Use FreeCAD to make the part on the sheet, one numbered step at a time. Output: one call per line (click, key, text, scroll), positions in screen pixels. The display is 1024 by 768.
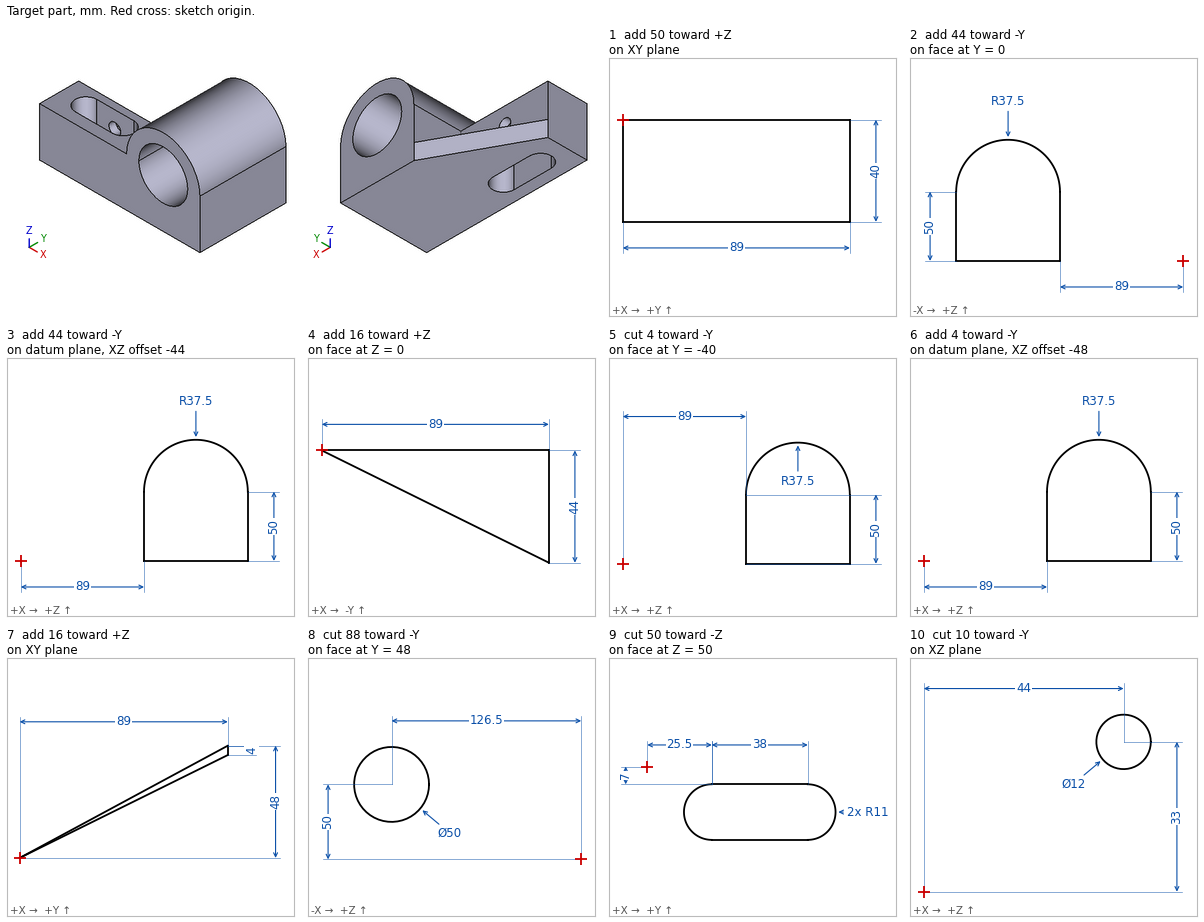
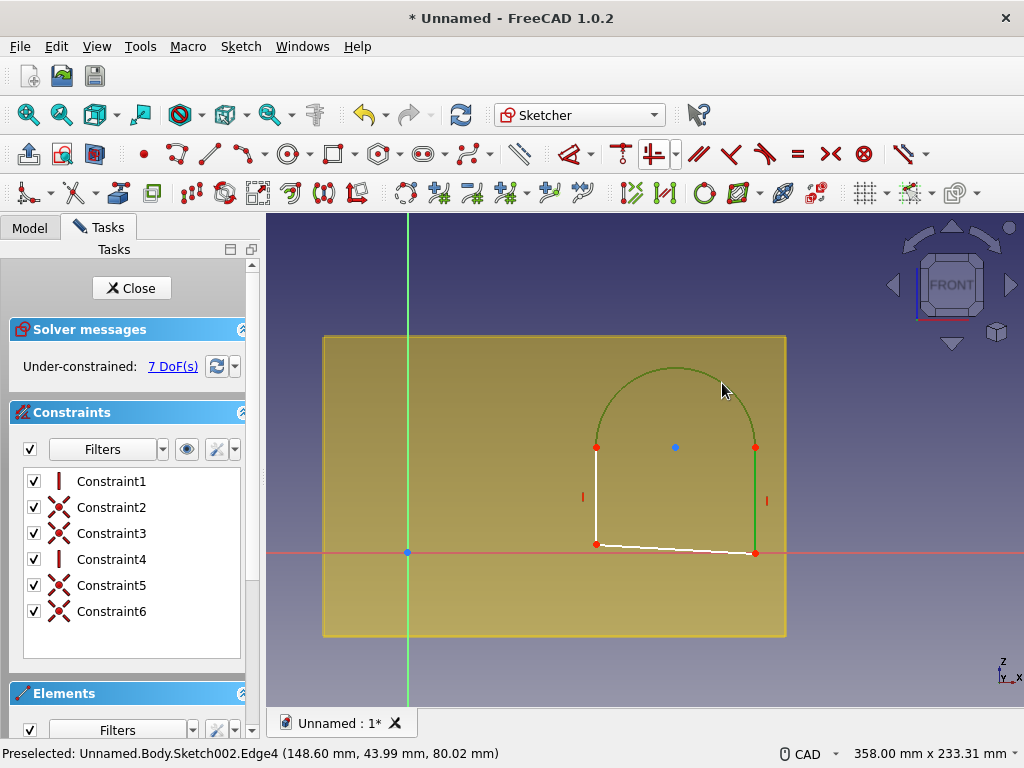
click(765, 154)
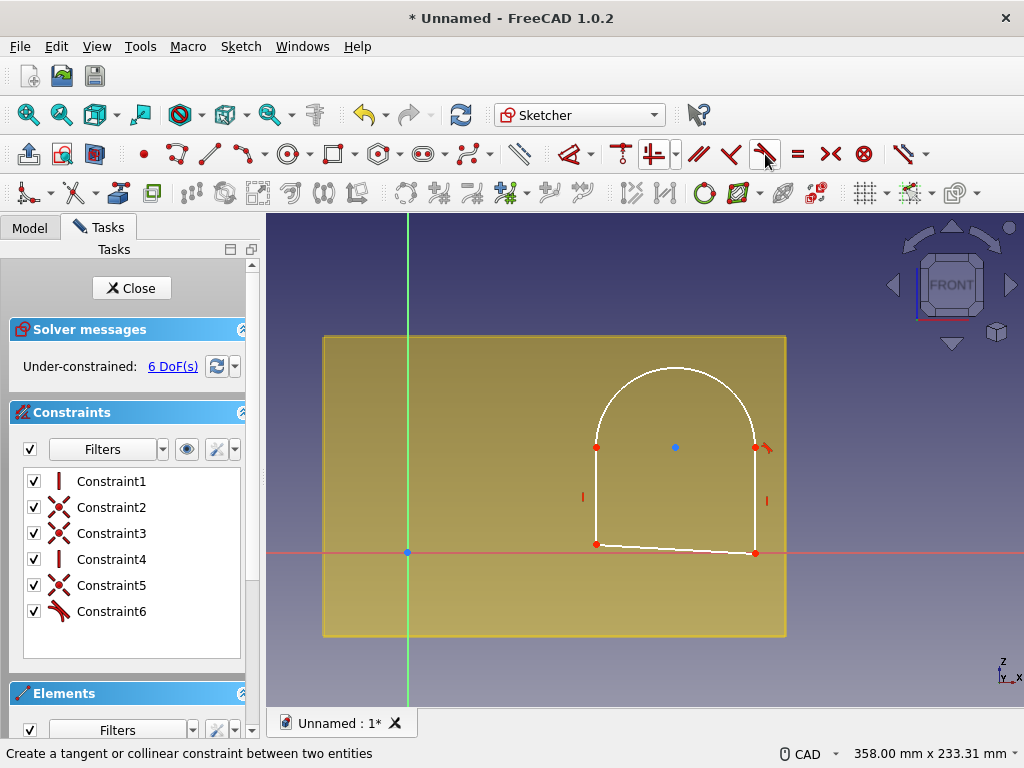
click(596, 516)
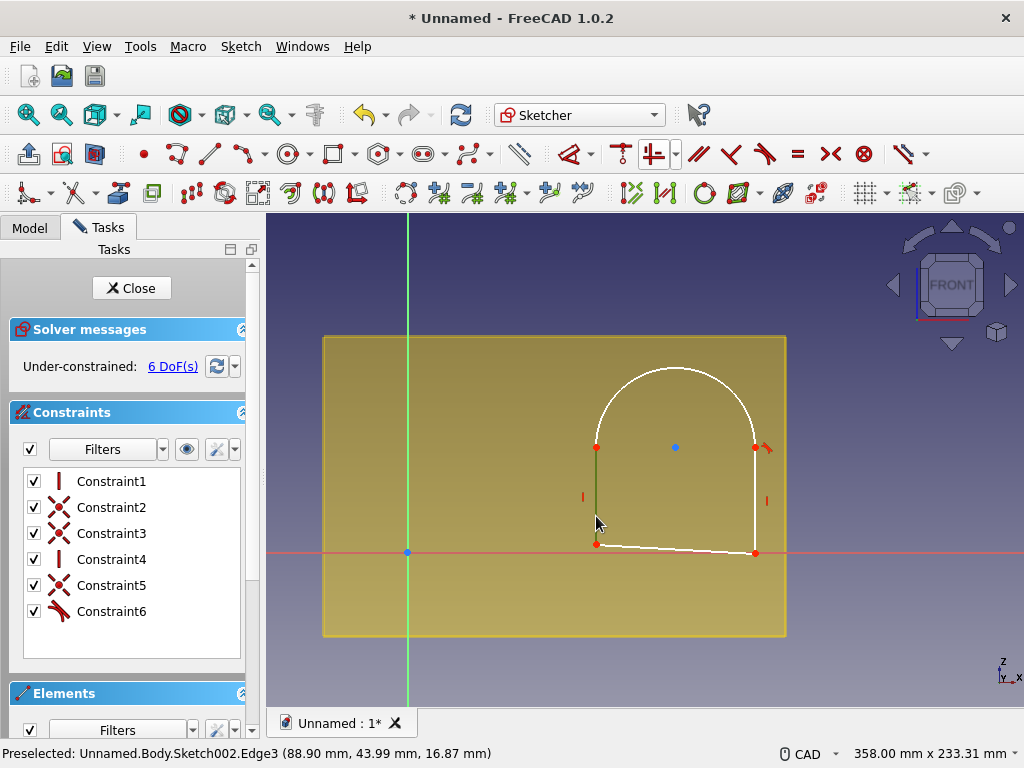
click(722, 383)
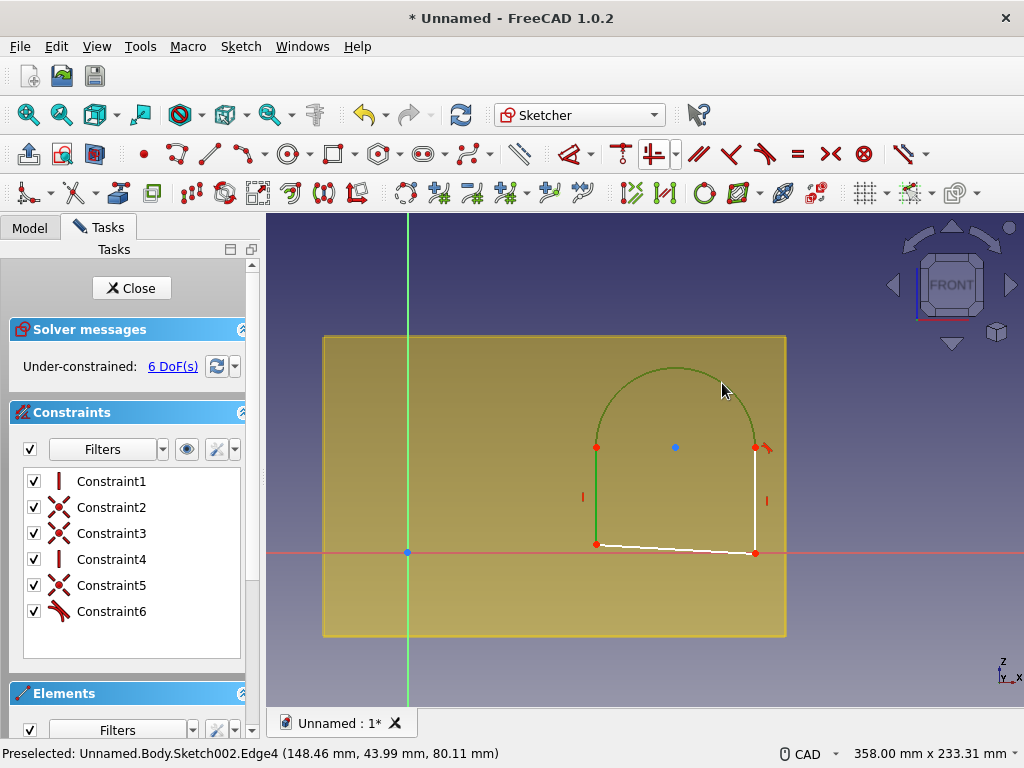
click(765, 154)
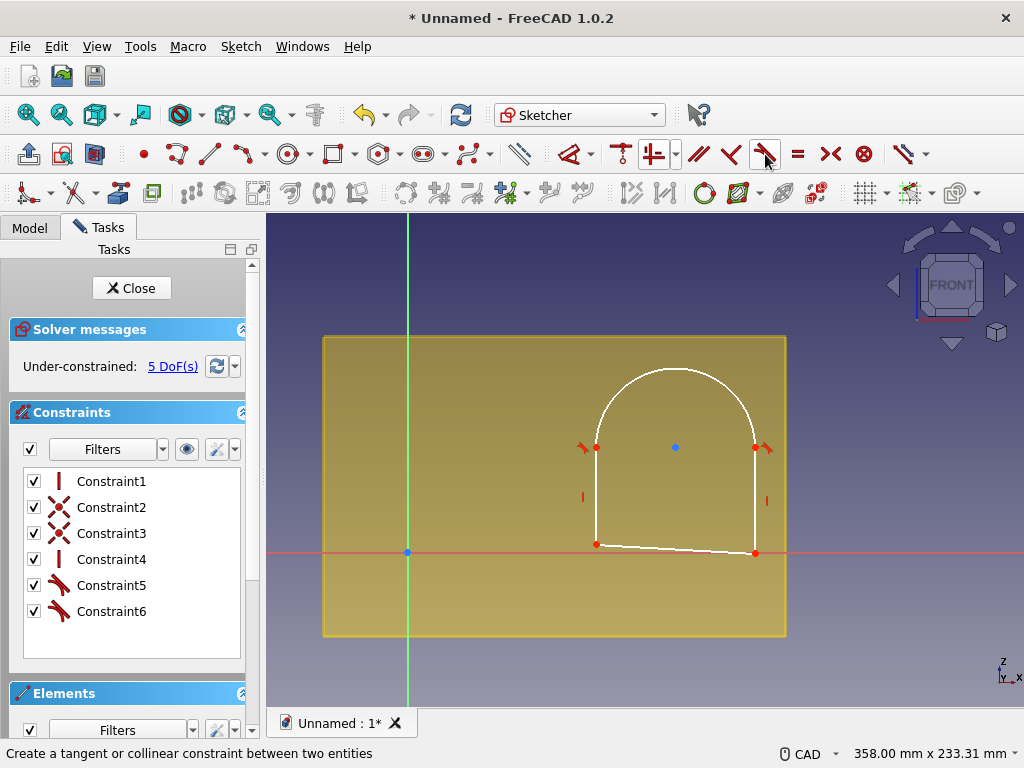
click(707, 551)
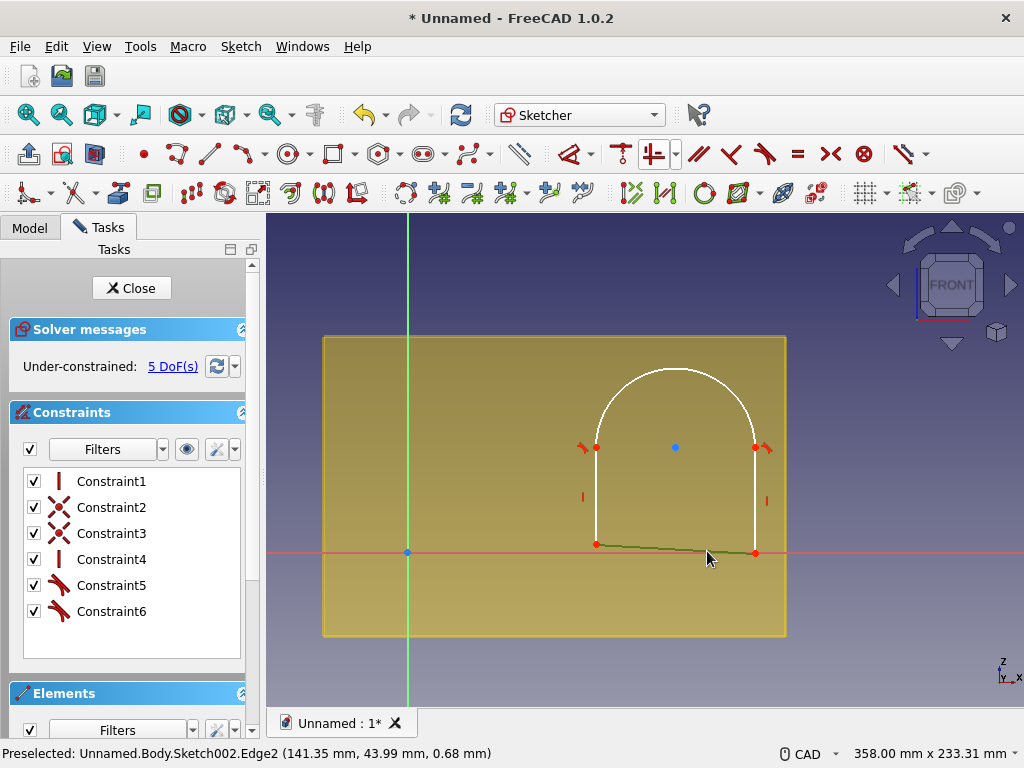
key(h)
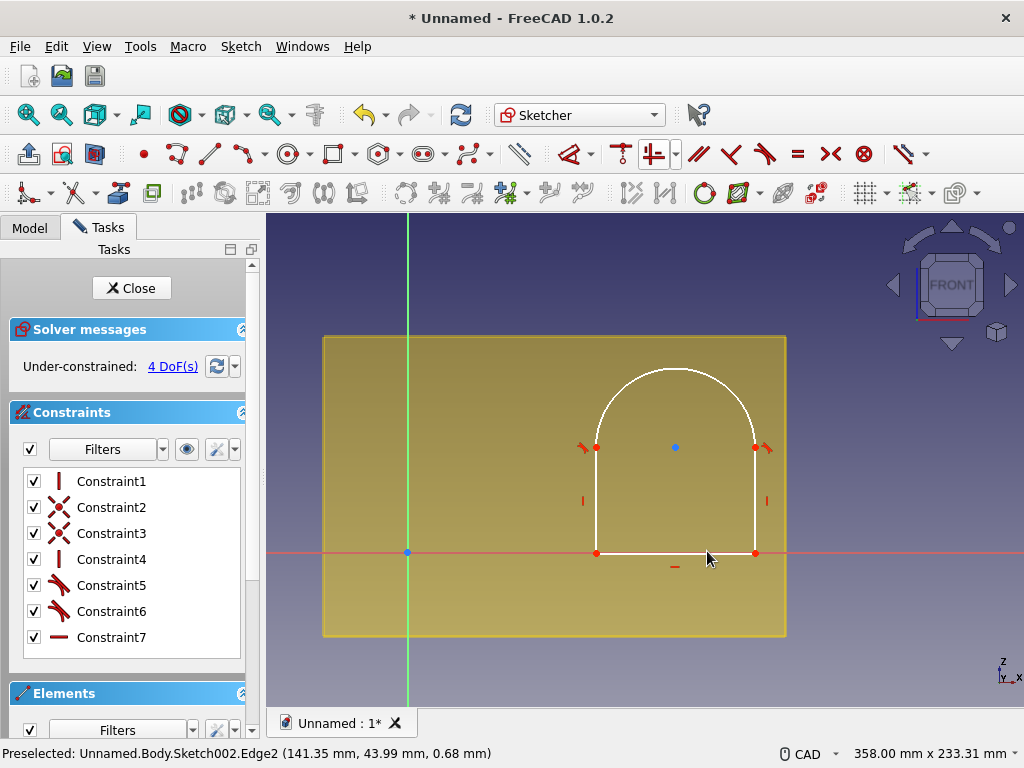
key(d)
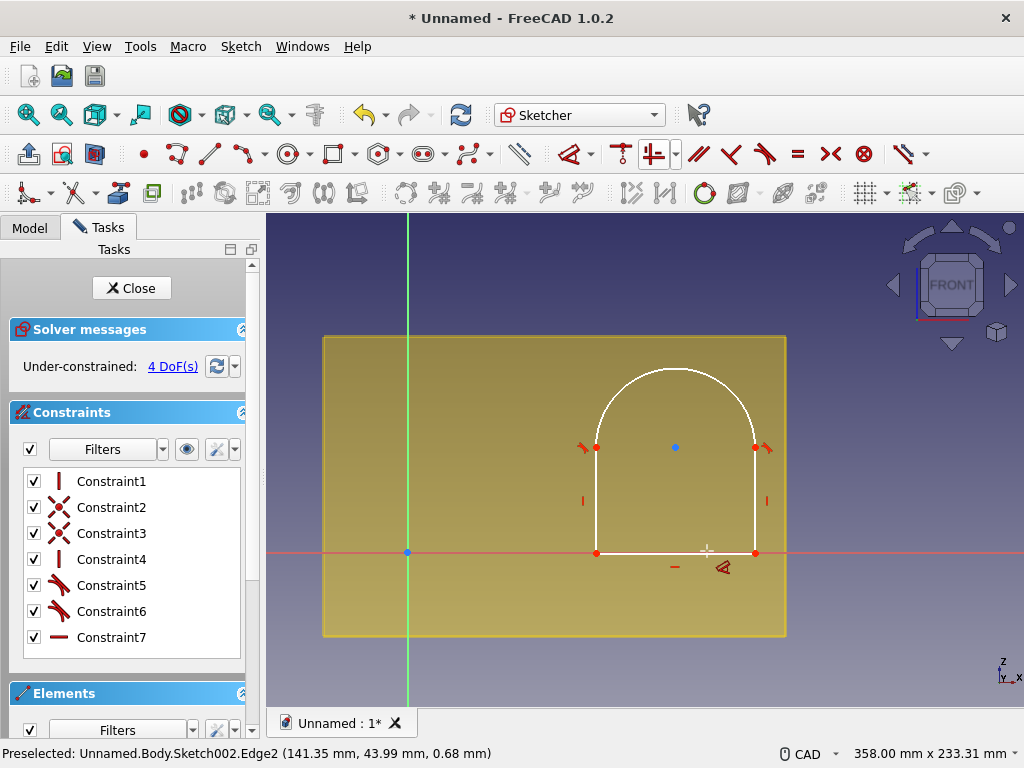
click(722, 384)
click(741, 358)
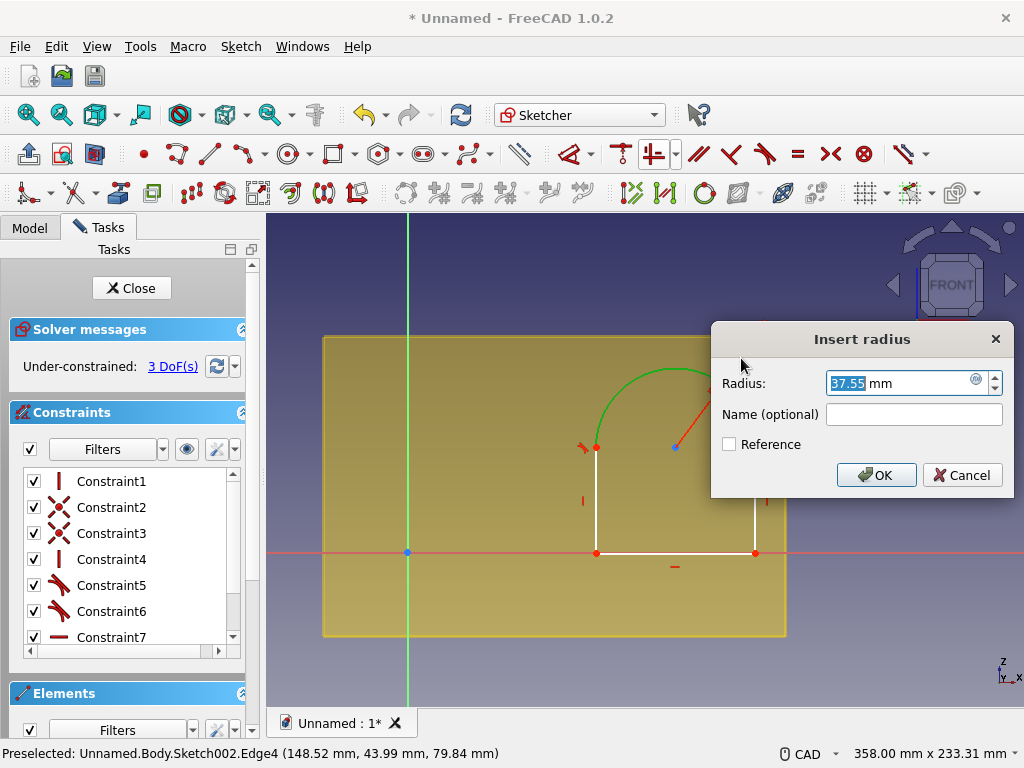
text(37.5)
key(Return)
key(Escape)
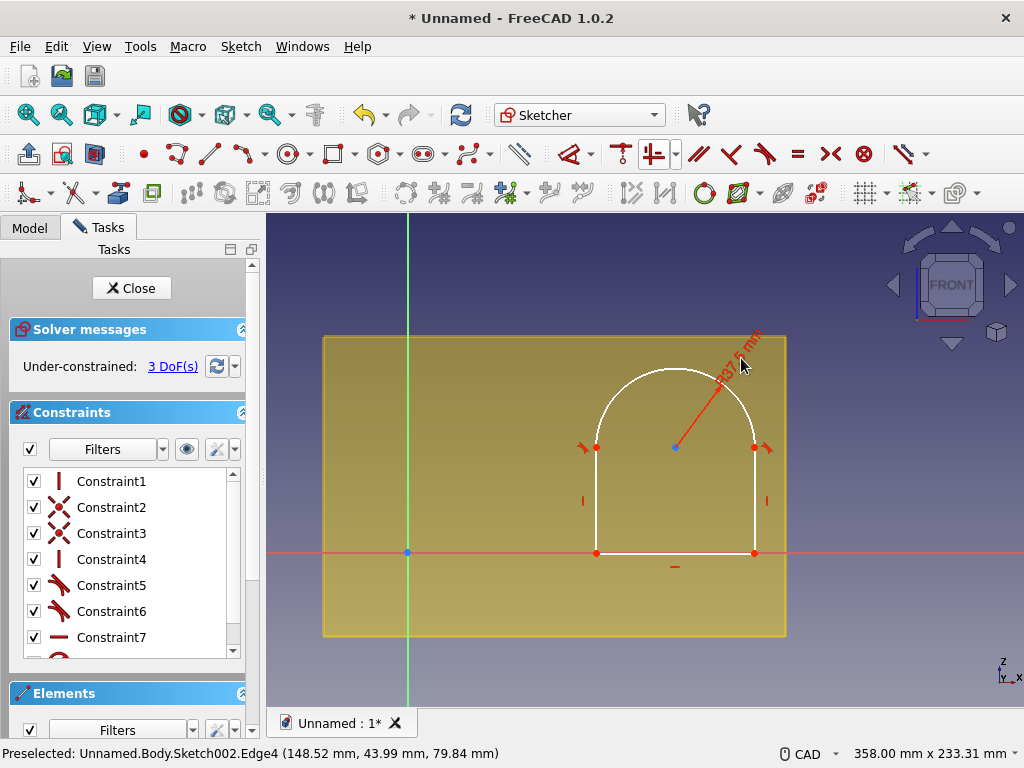
click(755, 554)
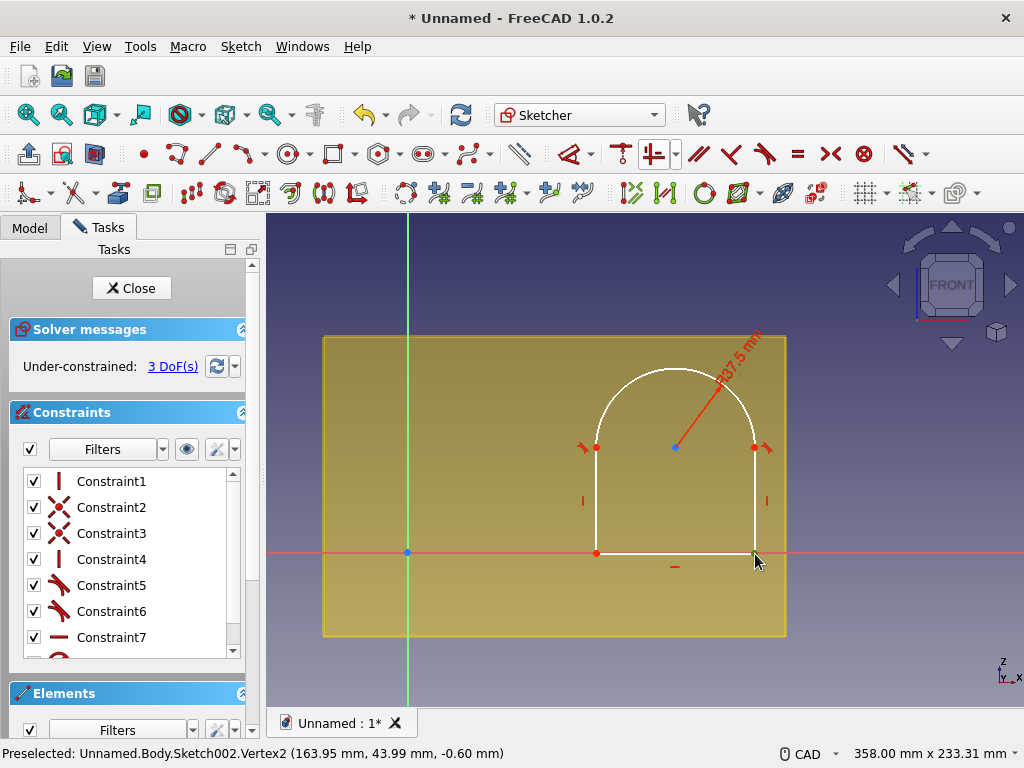
click(334, 553)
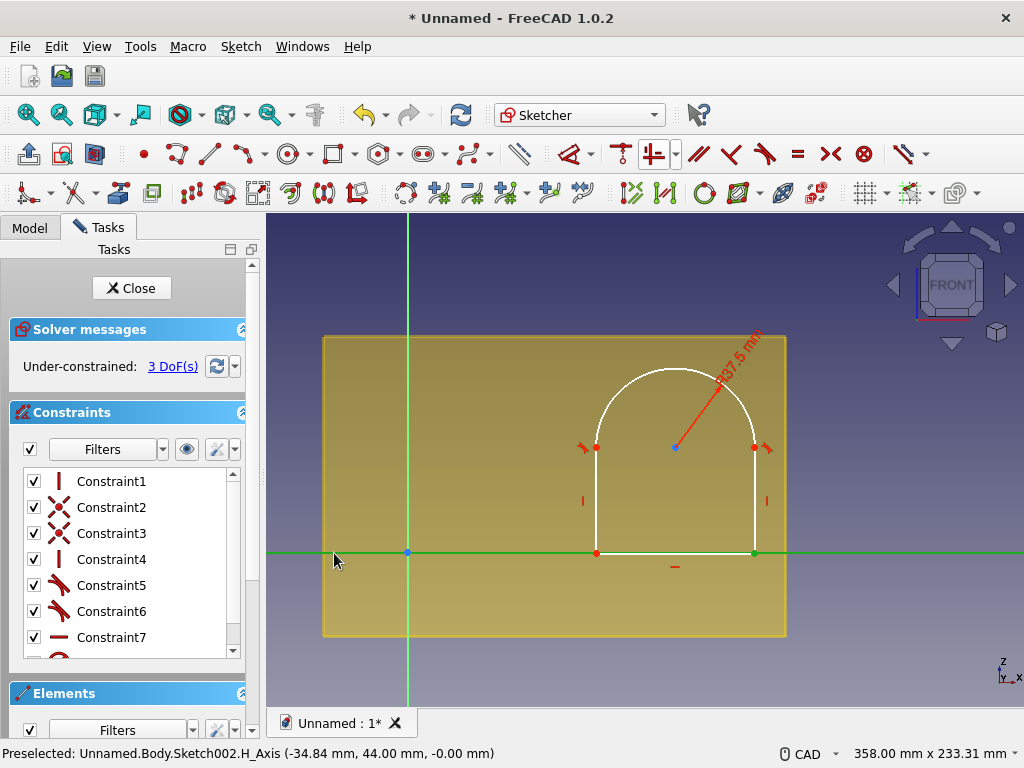
click(621, 154)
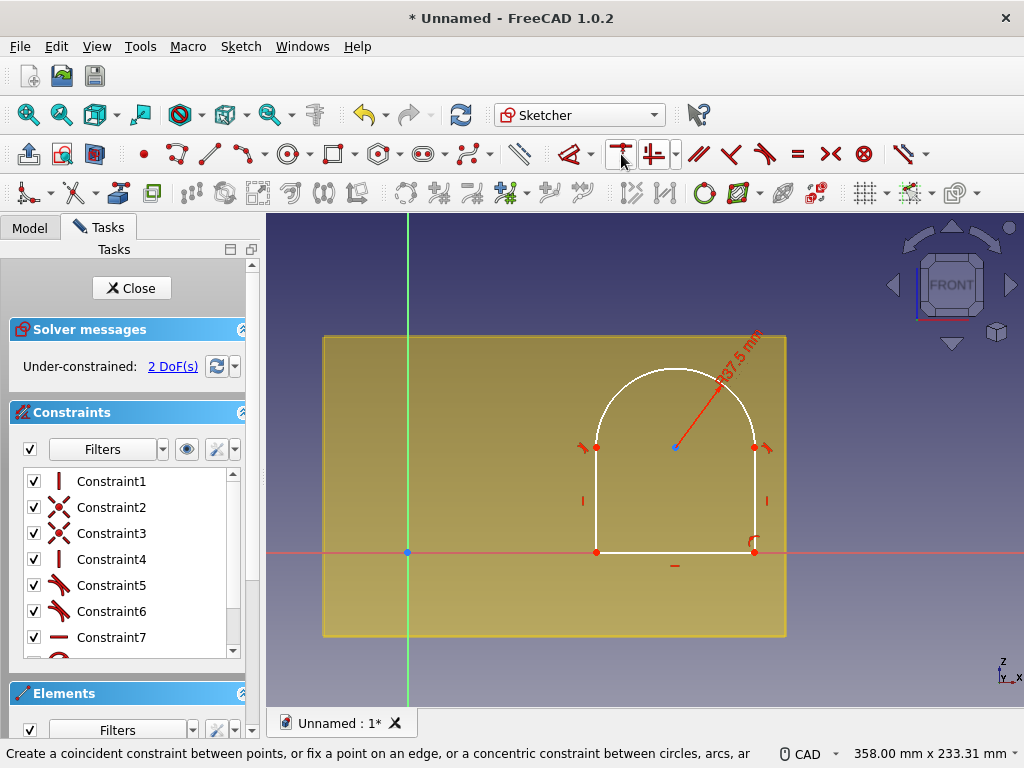
key(d)